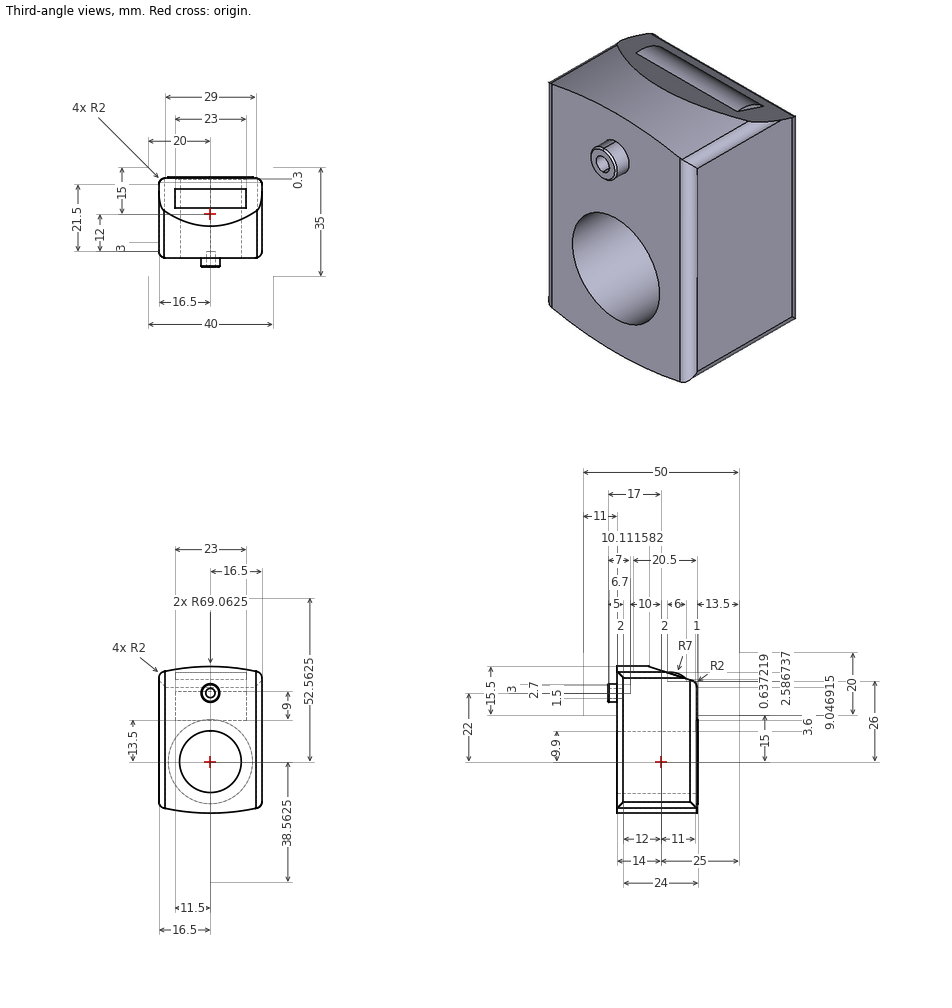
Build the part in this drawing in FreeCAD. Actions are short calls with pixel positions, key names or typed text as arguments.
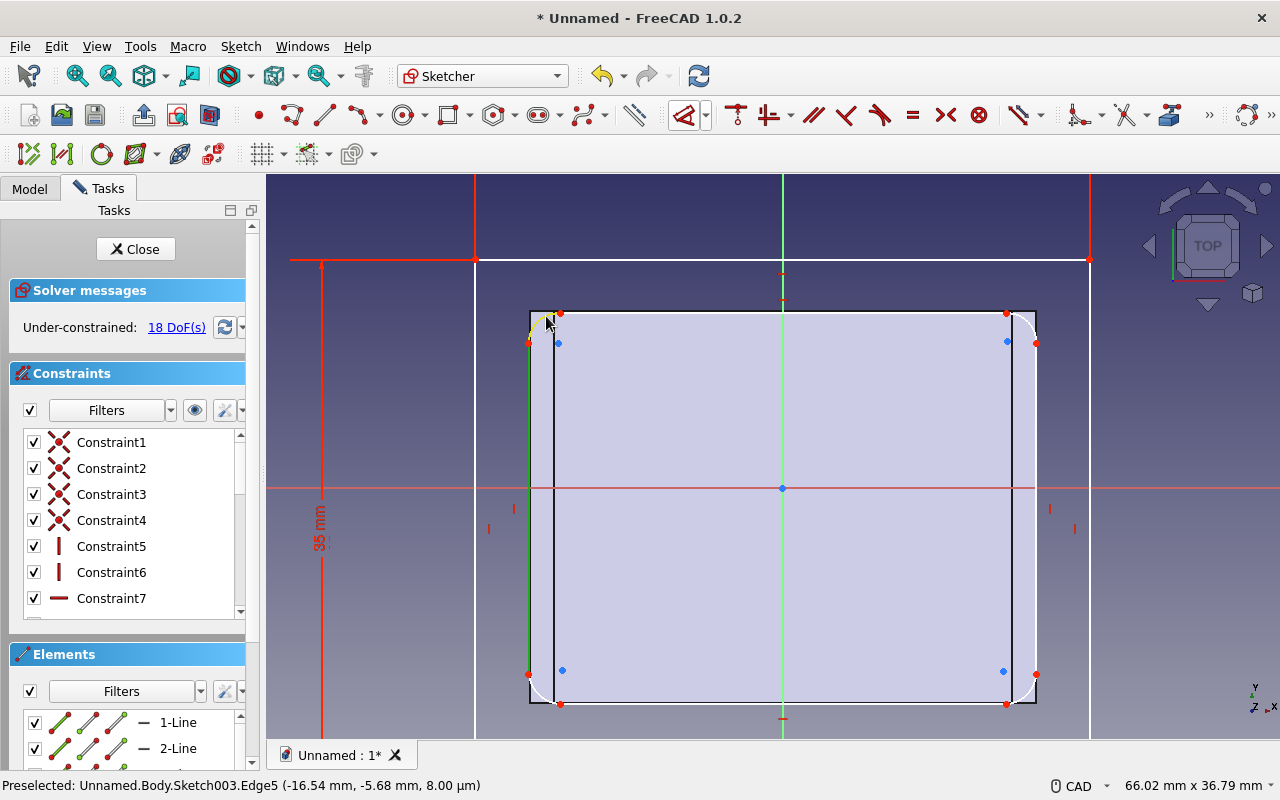
click(546, 316)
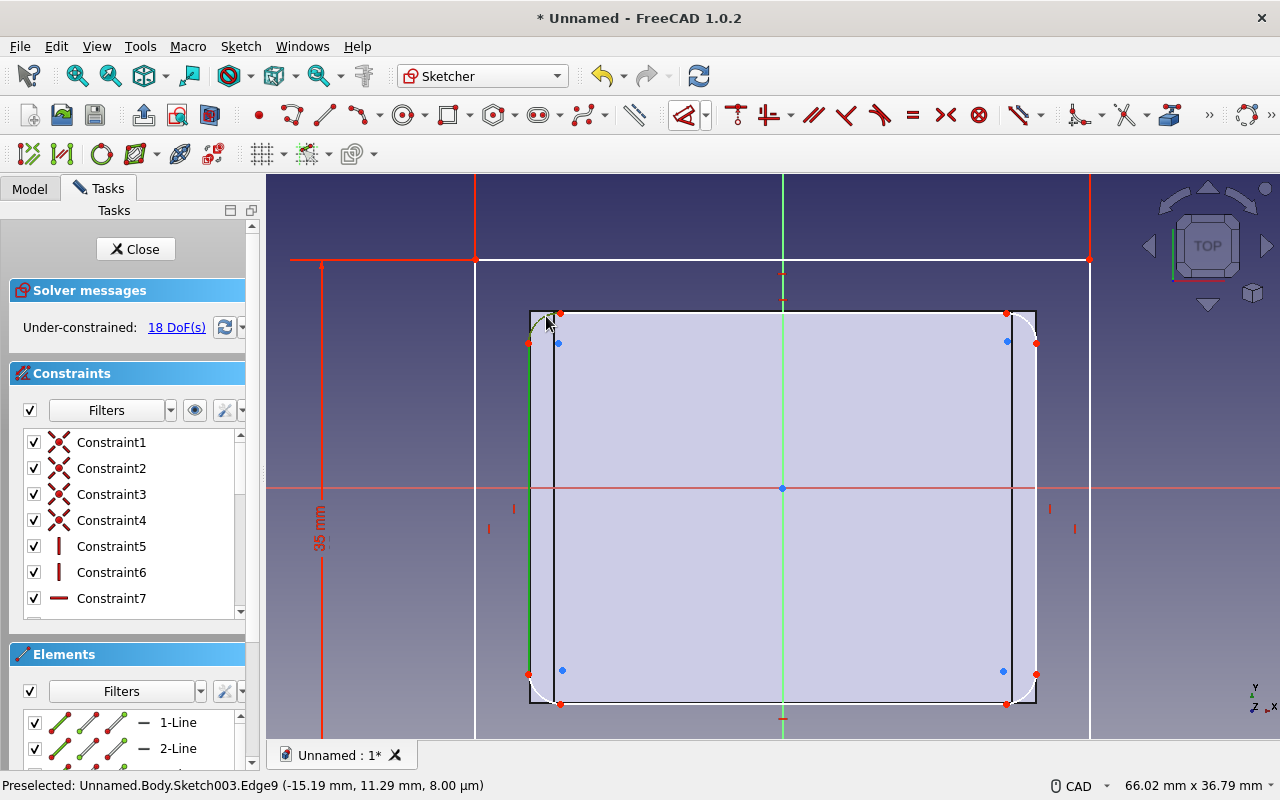
click(880, 116)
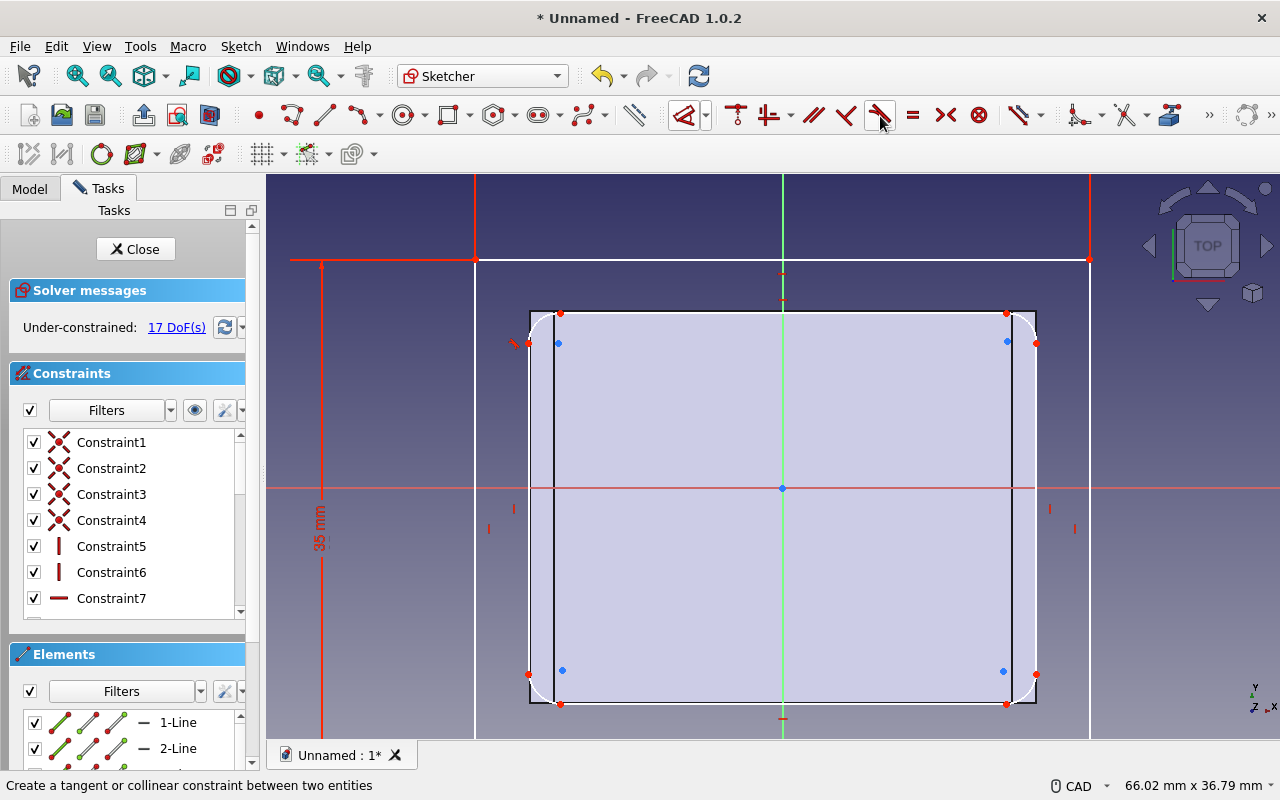
click(529, 575)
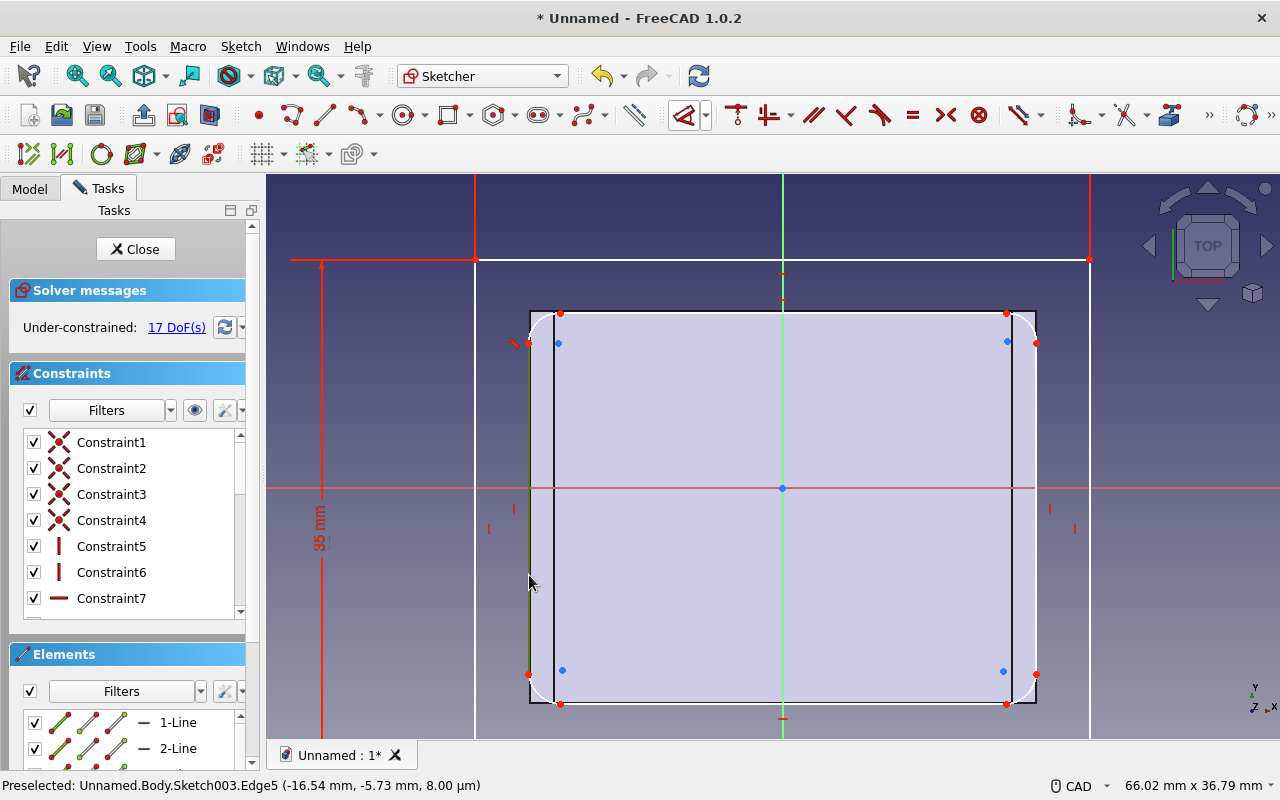
click(533, 688)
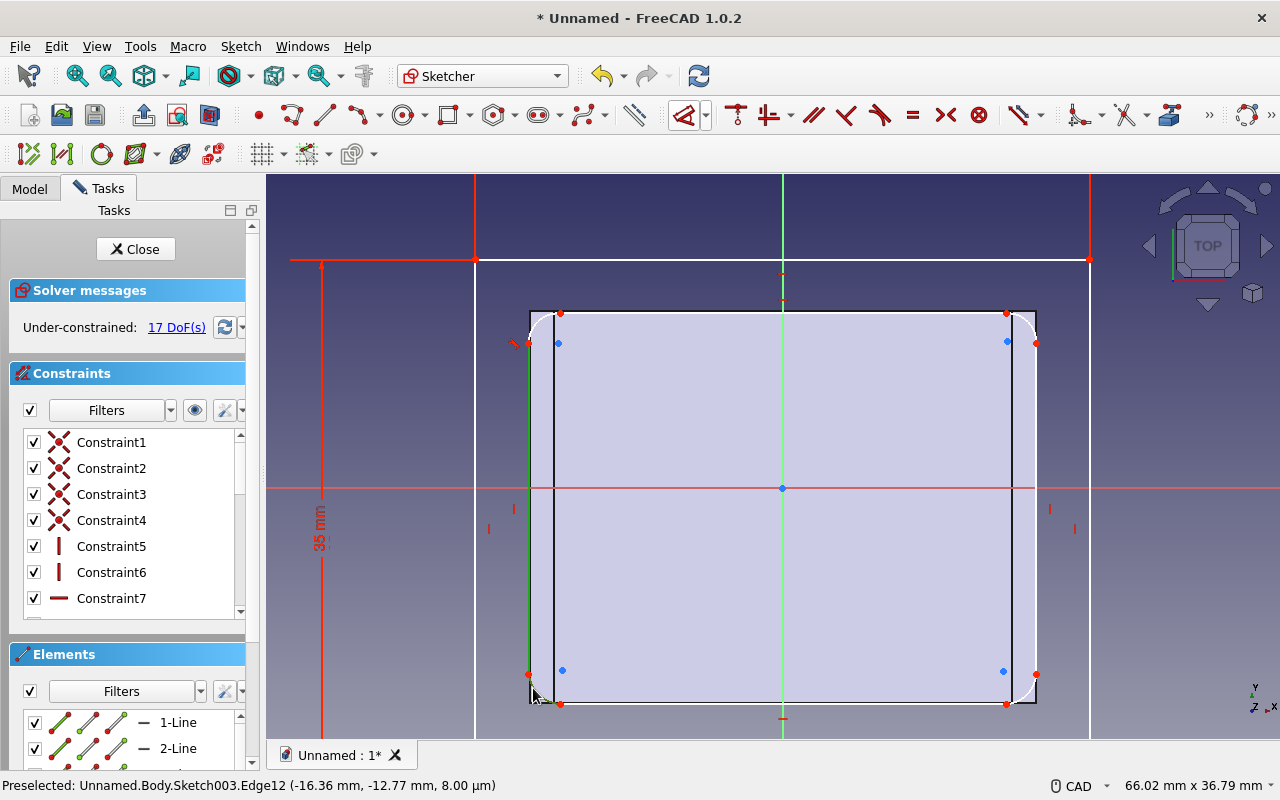
click(880, 116)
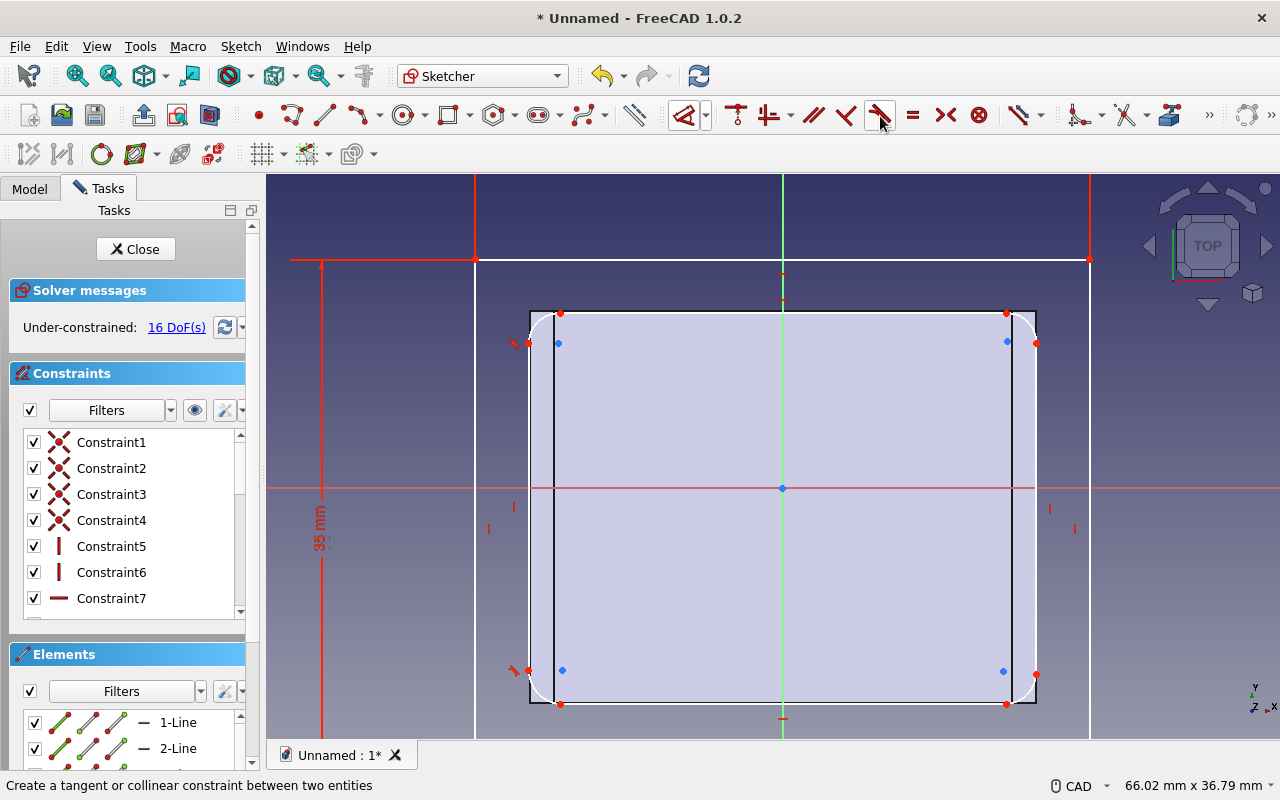
click(694, 313)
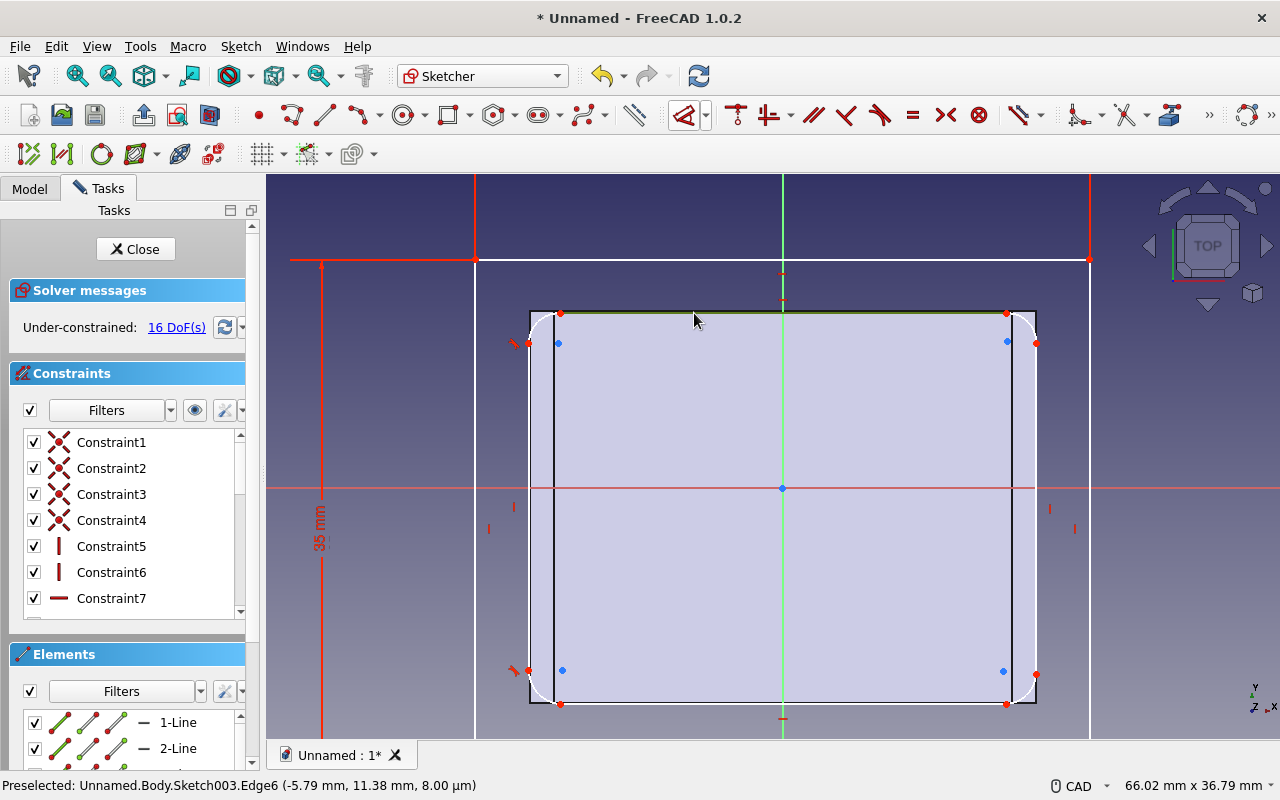
click(546, 316)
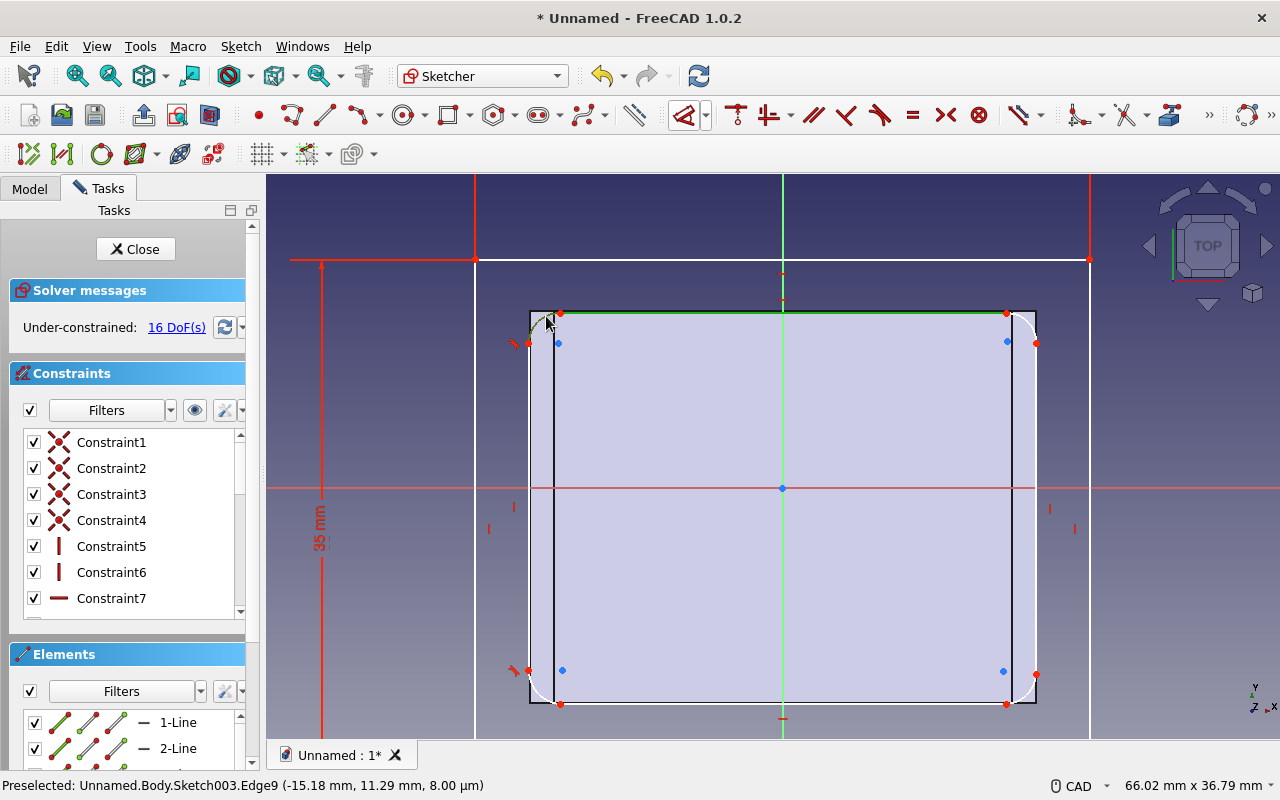
click(880, 116)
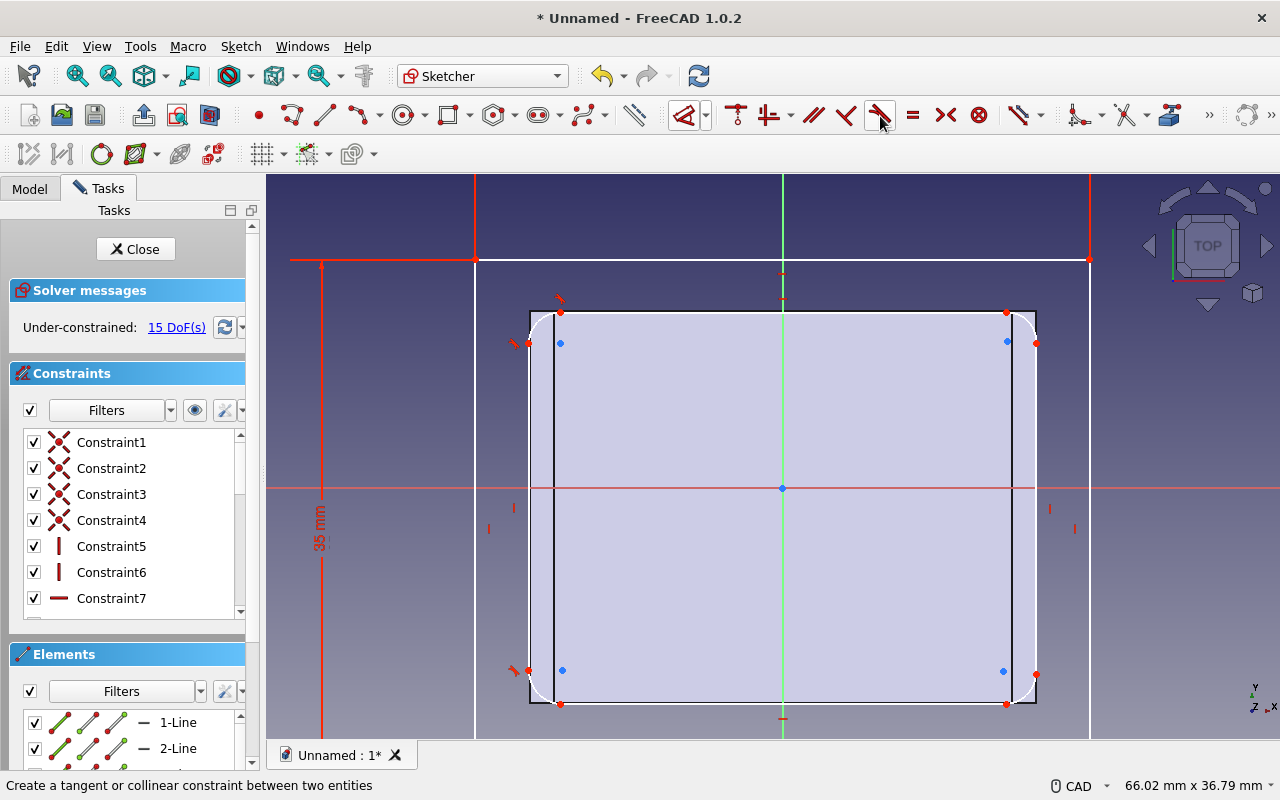
click(694, 313)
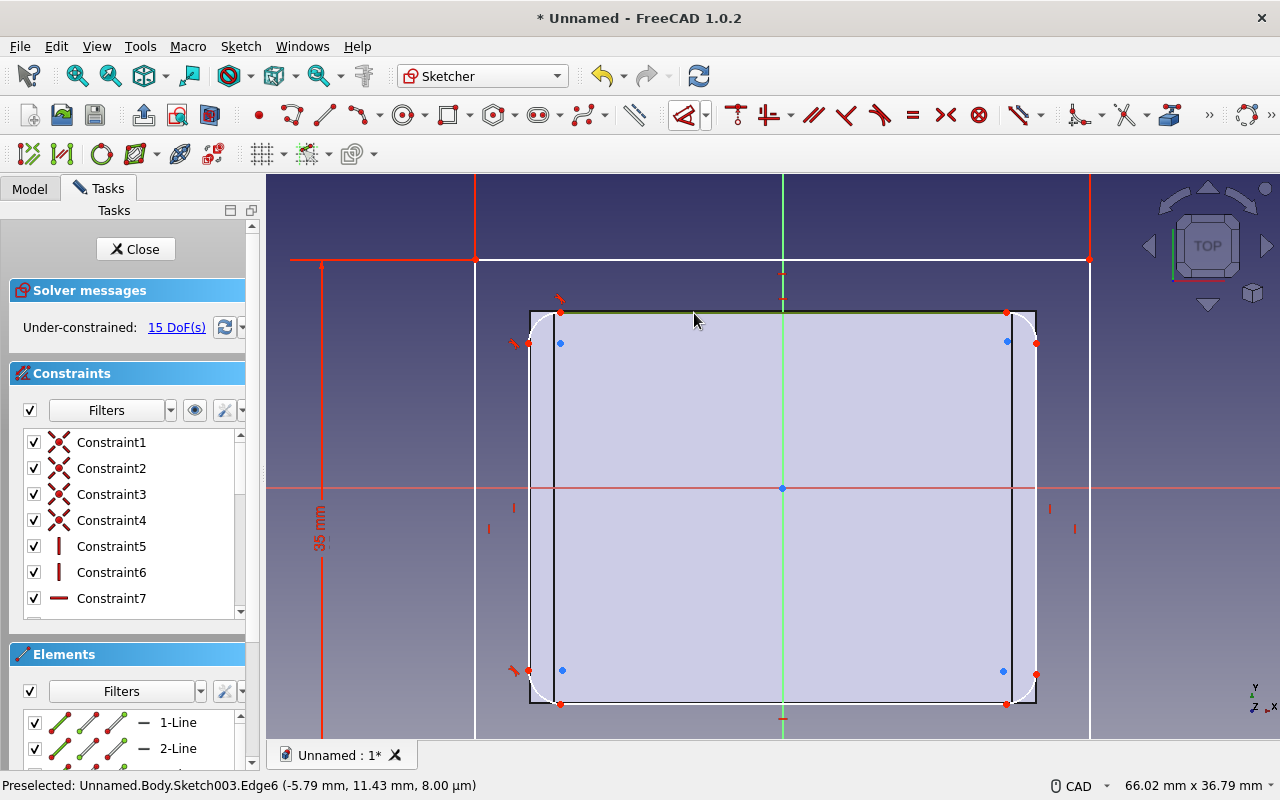
click(1033, 329)